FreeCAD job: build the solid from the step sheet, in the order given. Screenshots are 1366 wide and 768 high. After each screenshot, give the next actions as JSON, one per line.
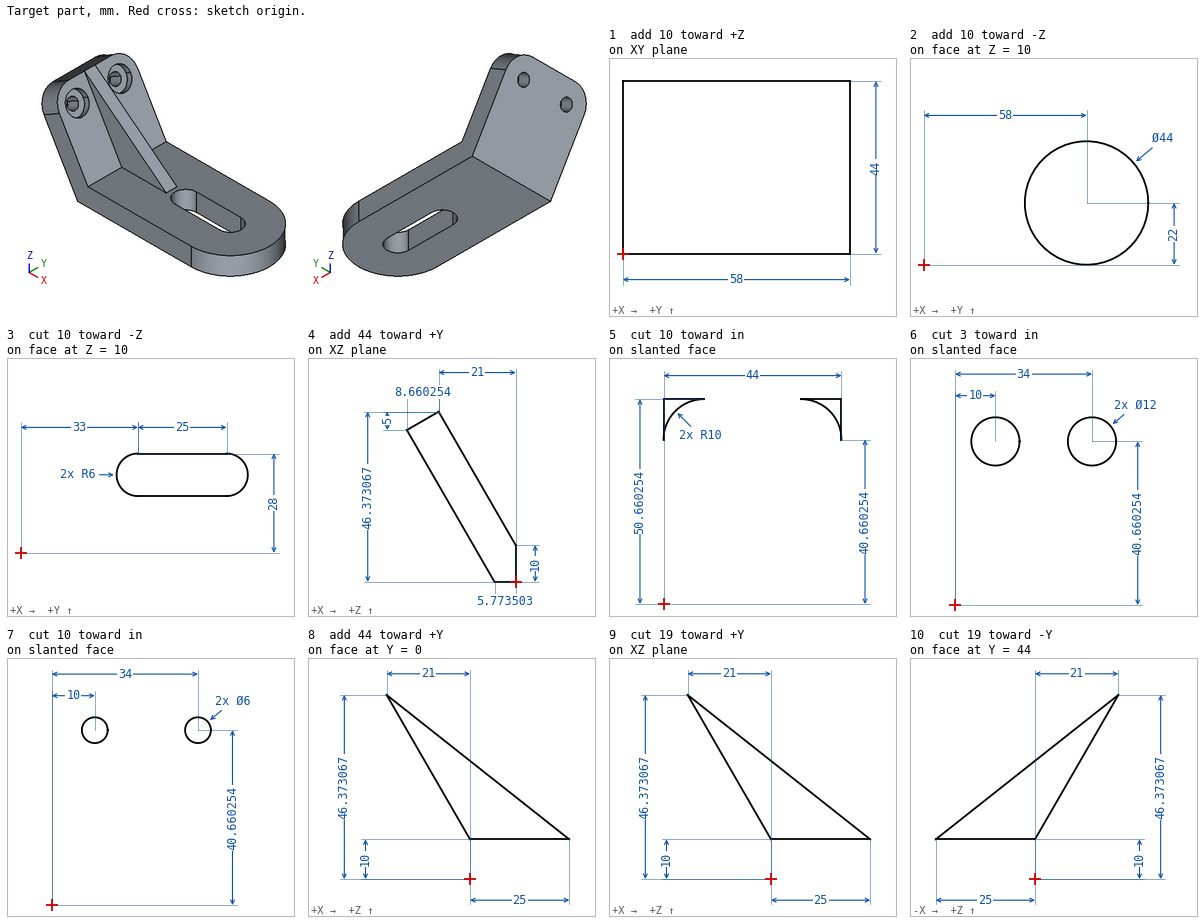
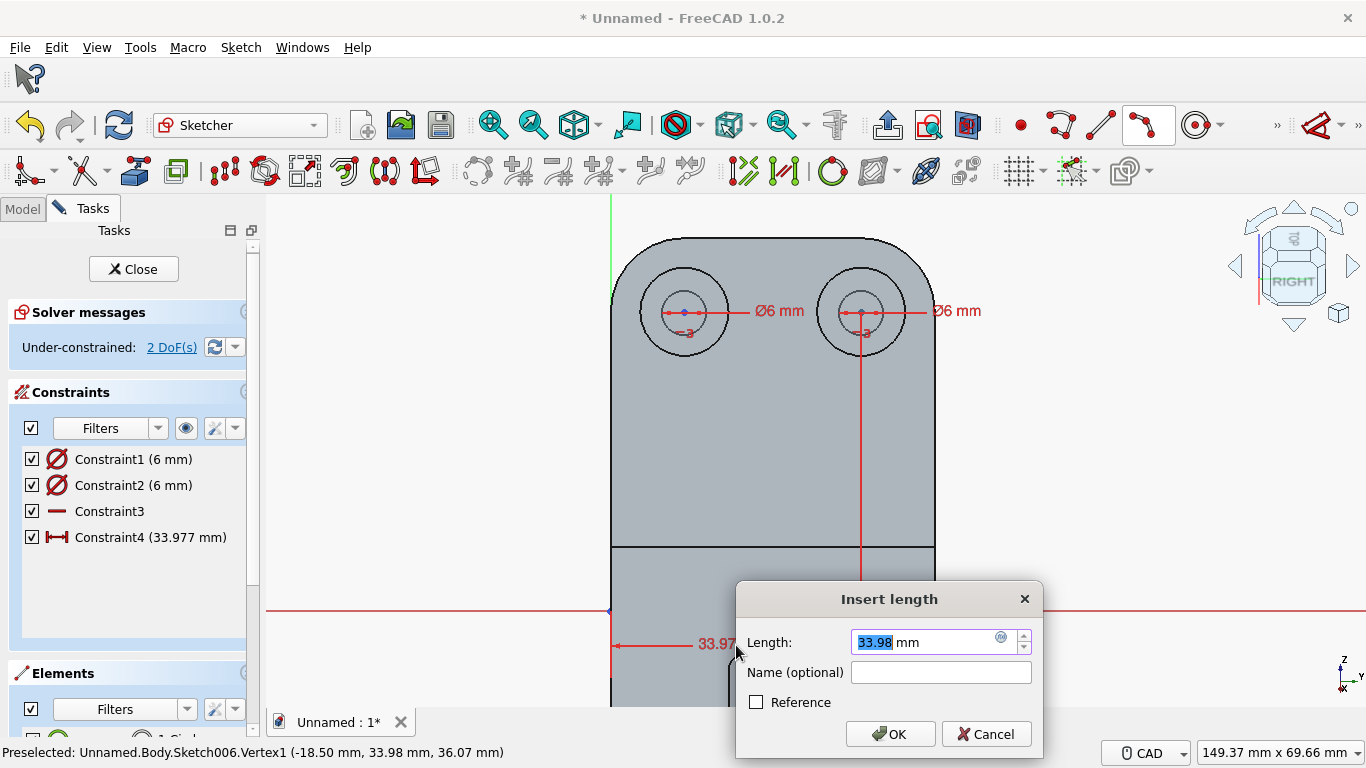
{"action": "type", "text": "34"}
{"action": "key", "text": "Return"}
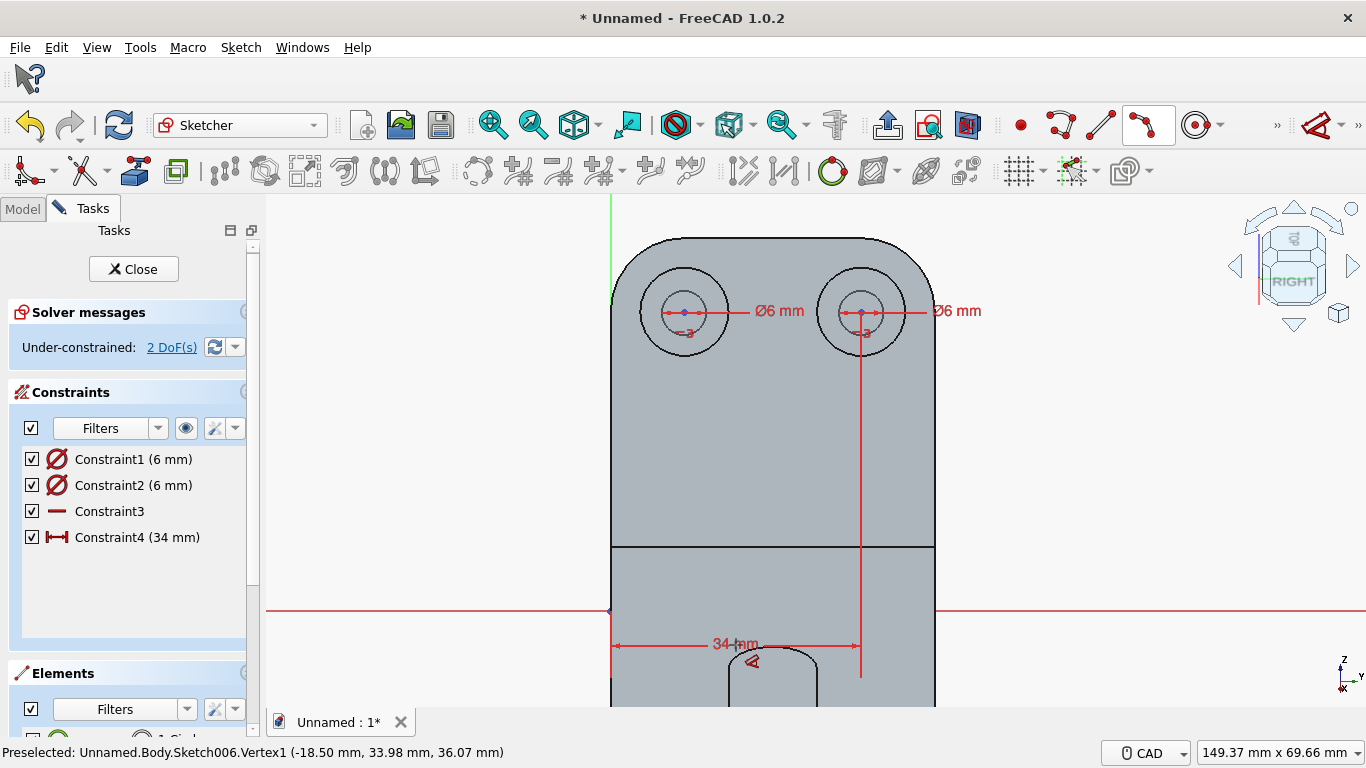
{"action": "left_click", "coordinate": [684, 313]}
{"action": "left_click", "coordinate": [647, 645]}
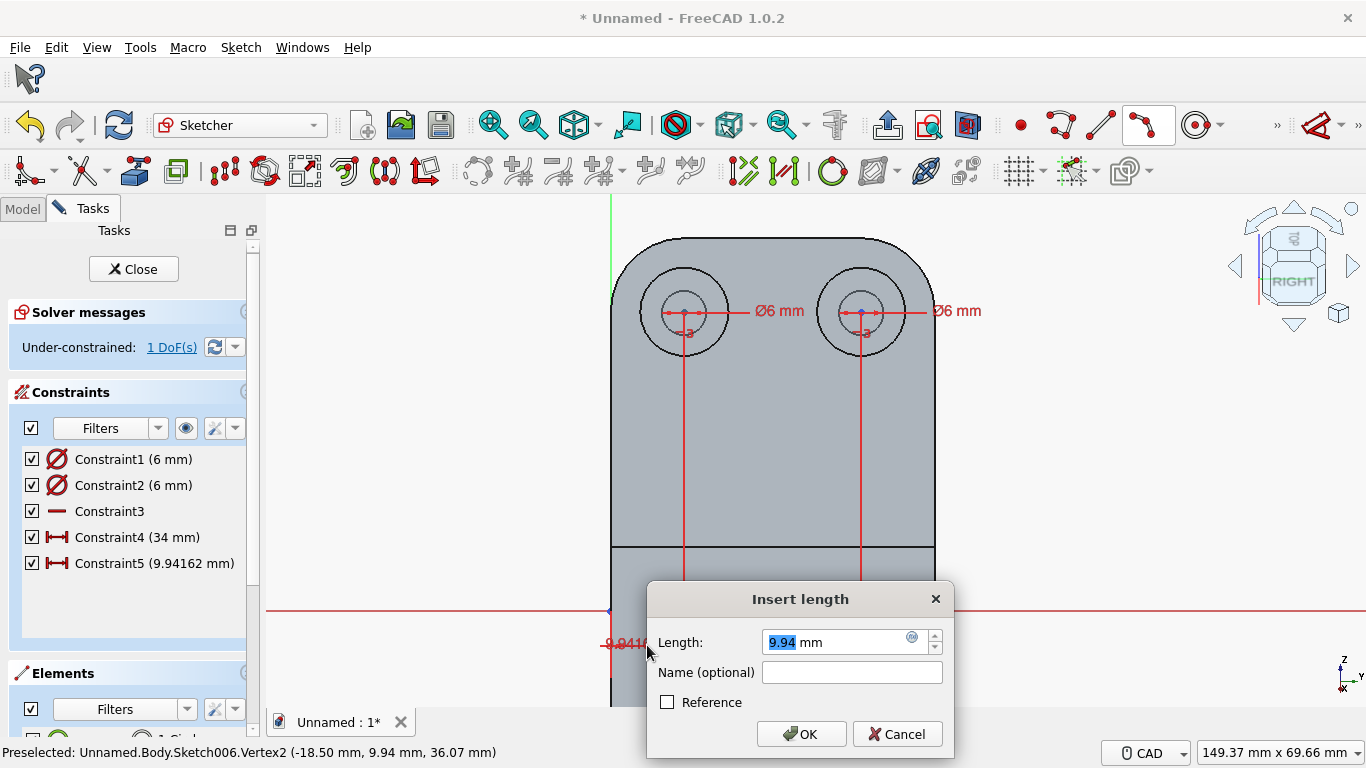
{"action": "type", "text": "10"}
{"action": "key", "text": "Return"}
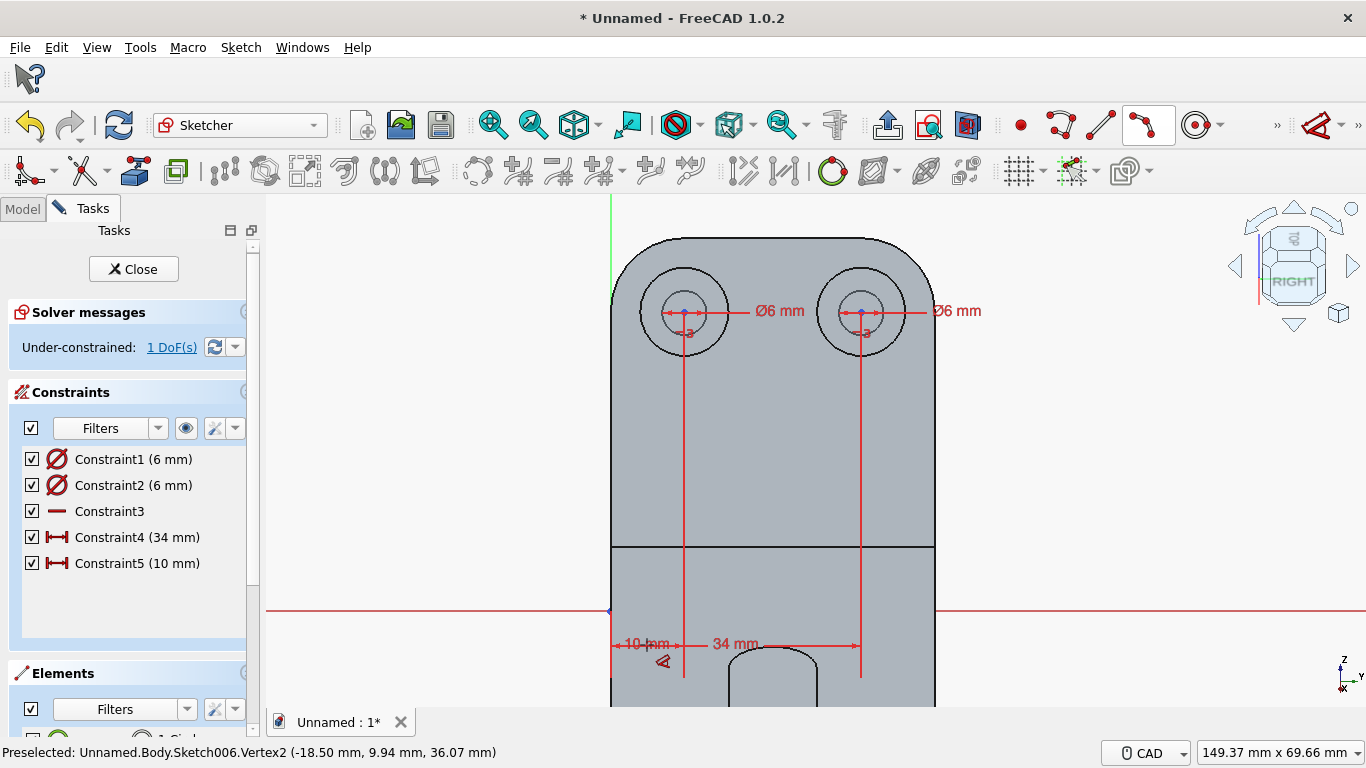
{"action": "left_click", "coordinate": [861, 313]}
{"action": "left_click", "coordinate": [577, 462]}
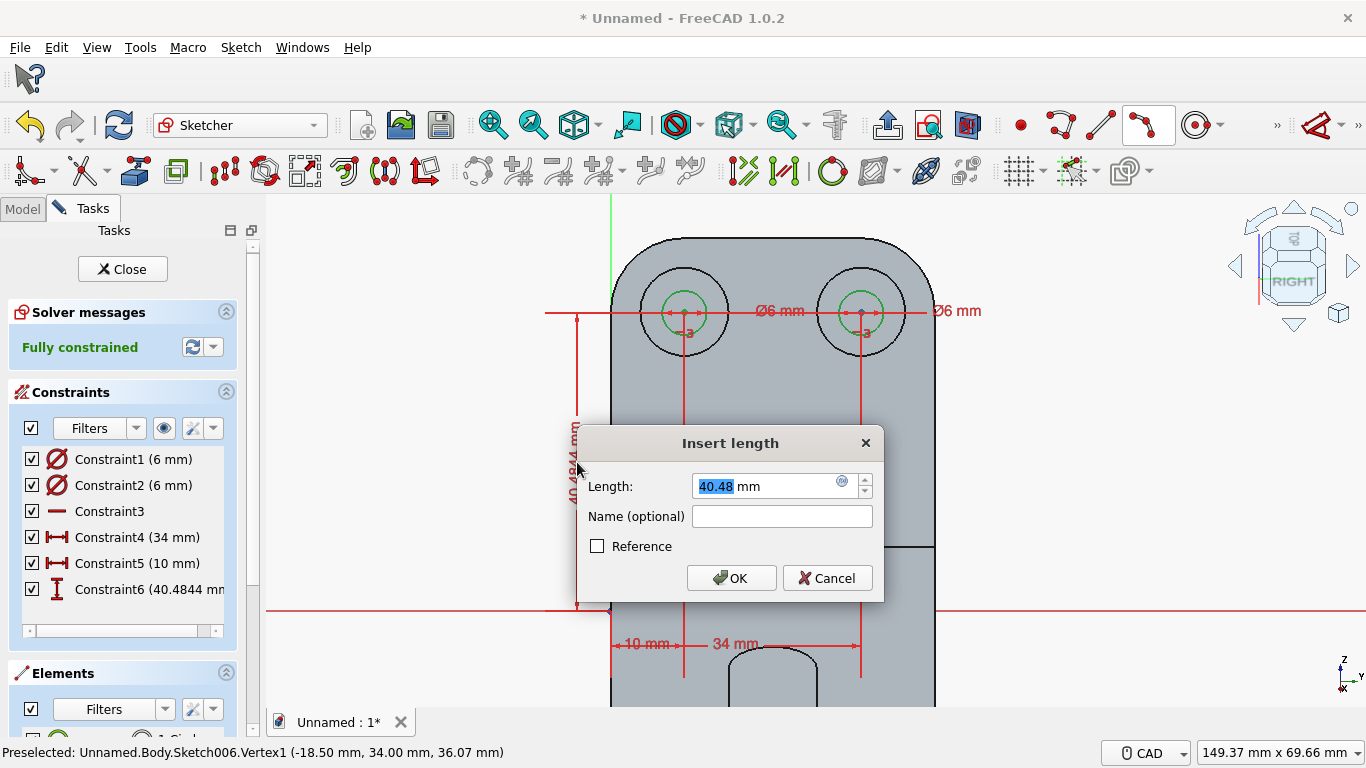
{"action": "type", "text": "40.660254"}
{"action": "key", "text": "Return"}
{"action": "key", "text": "Escape"}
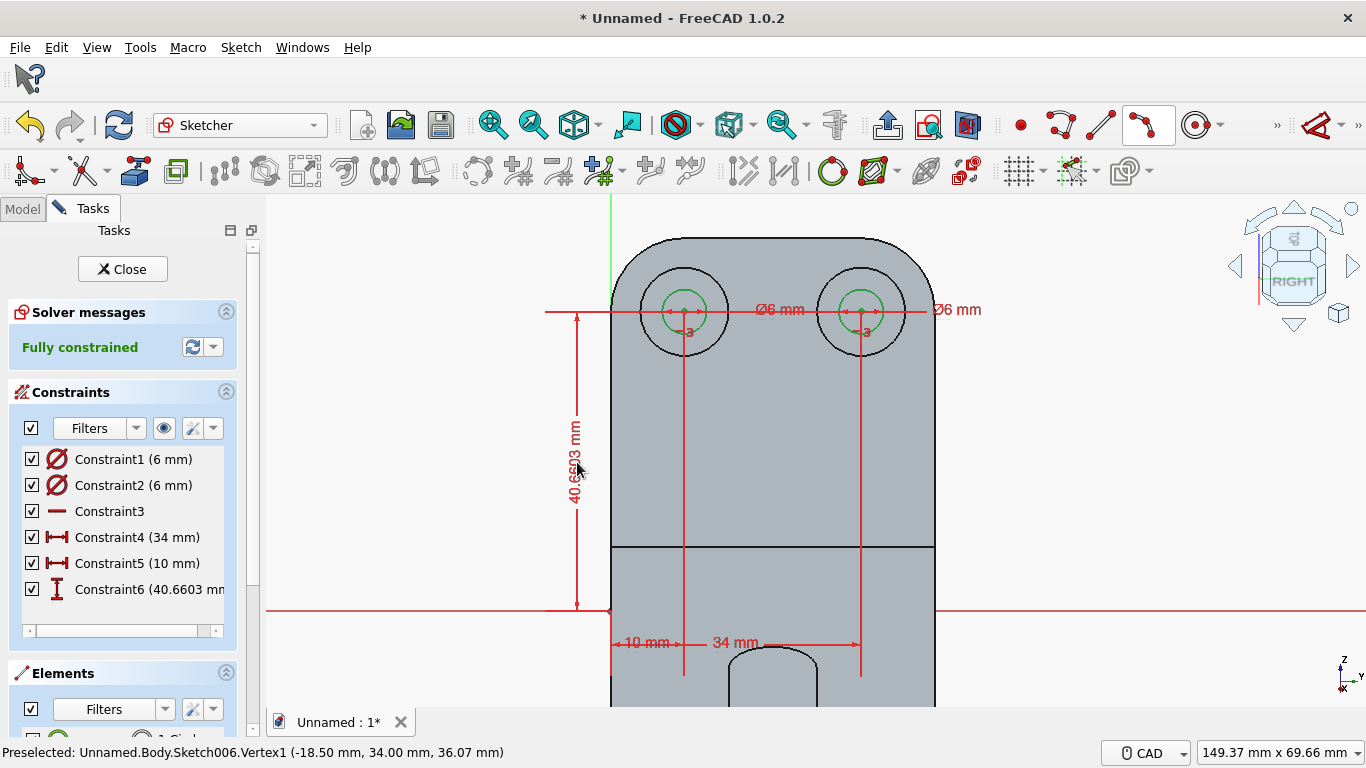
{"action": "left_click", "coordinate": [123, 269]}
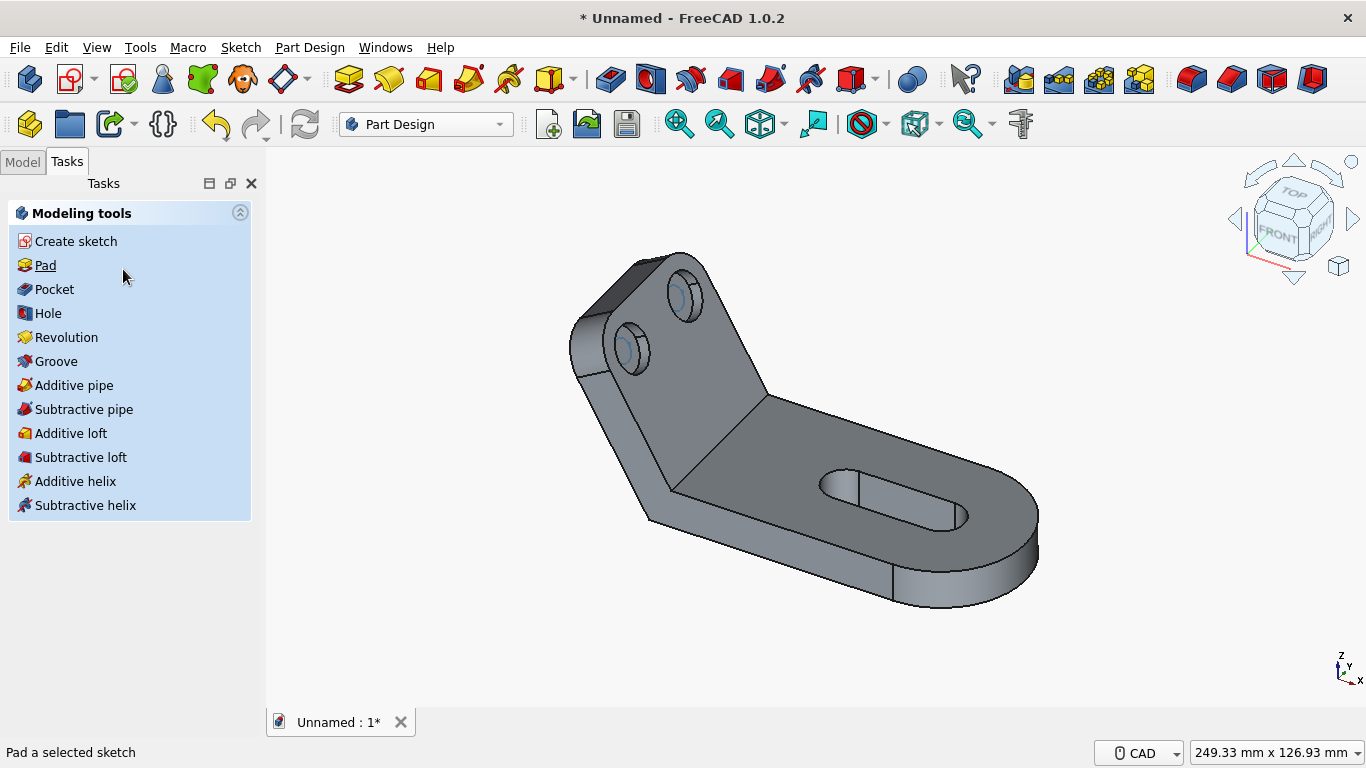
{"action": "left_click", "coordinate": [612, 80]}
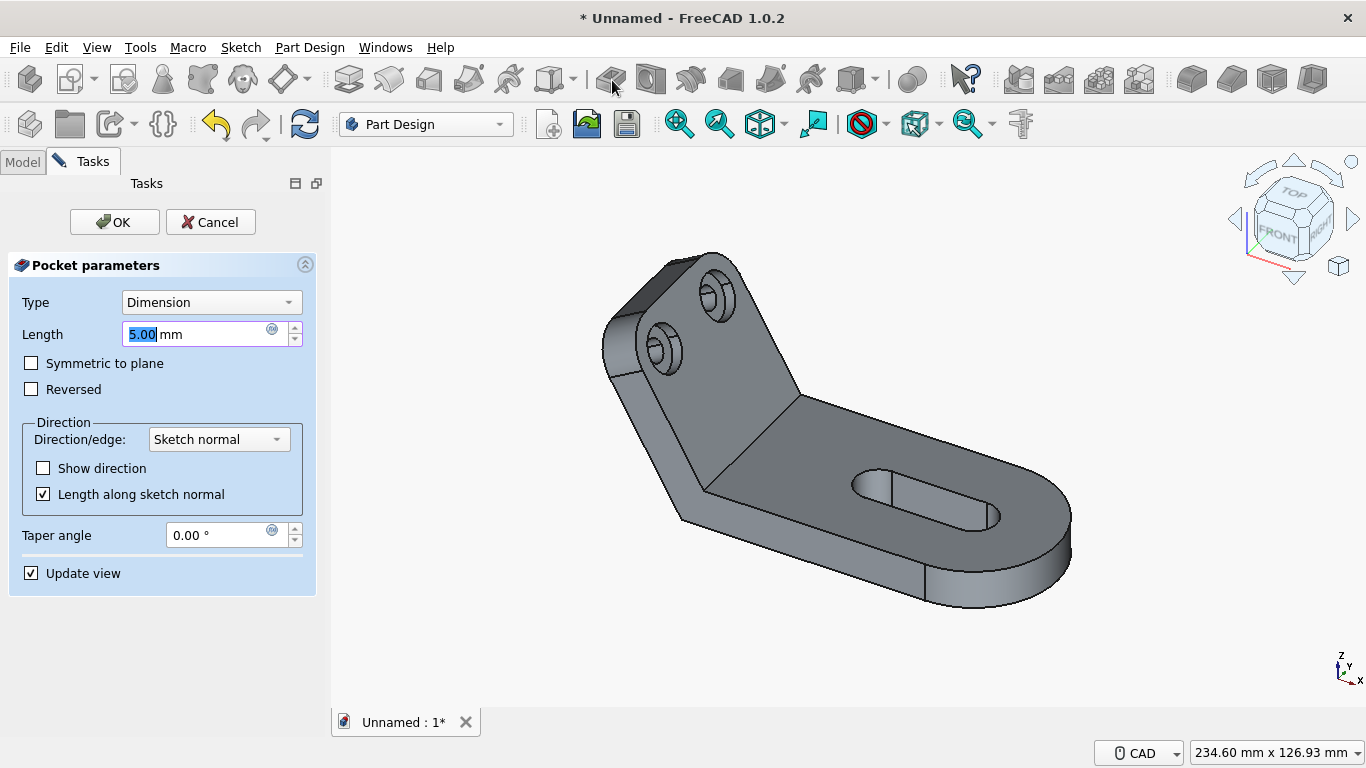
{"action": "type", "text": "10"}
{"action": "key", "text": "Tab"}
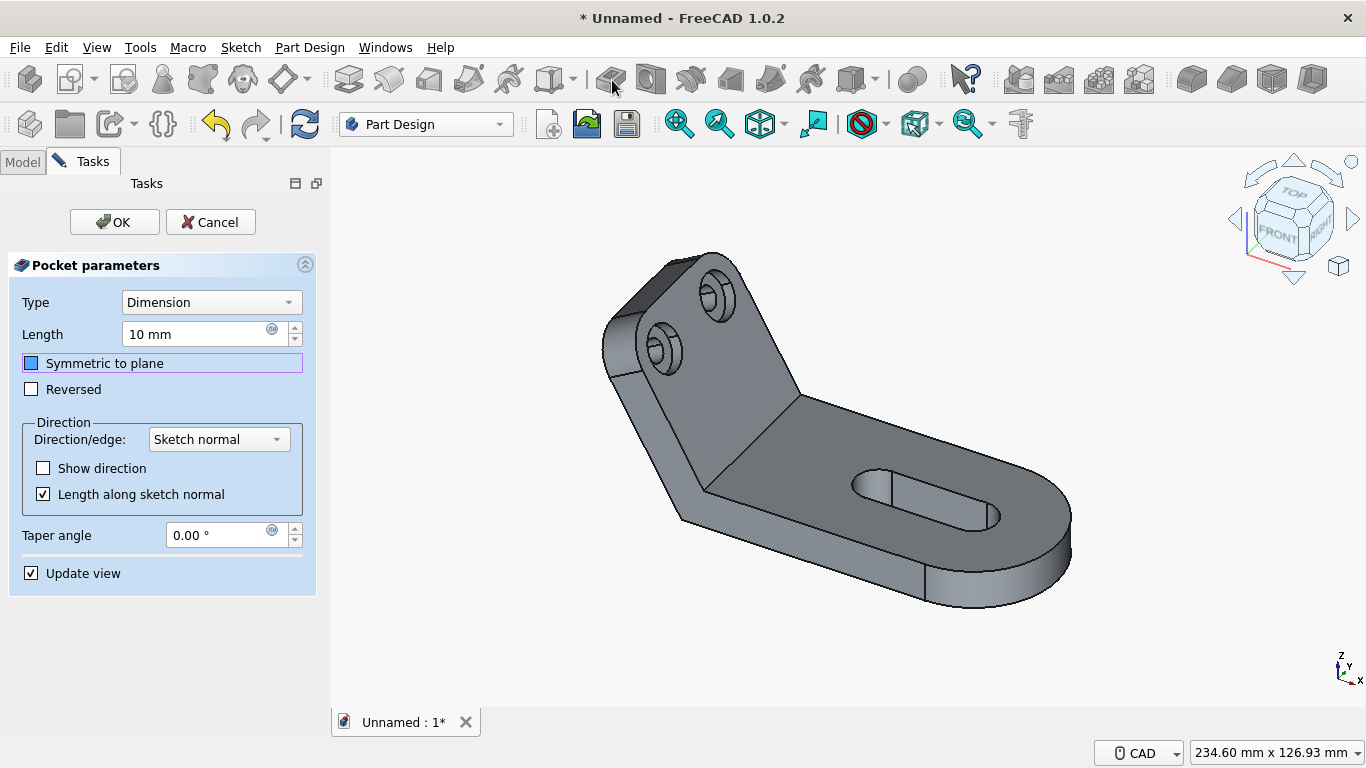
{"action": "left_click", "coordinate": [115, 222]}